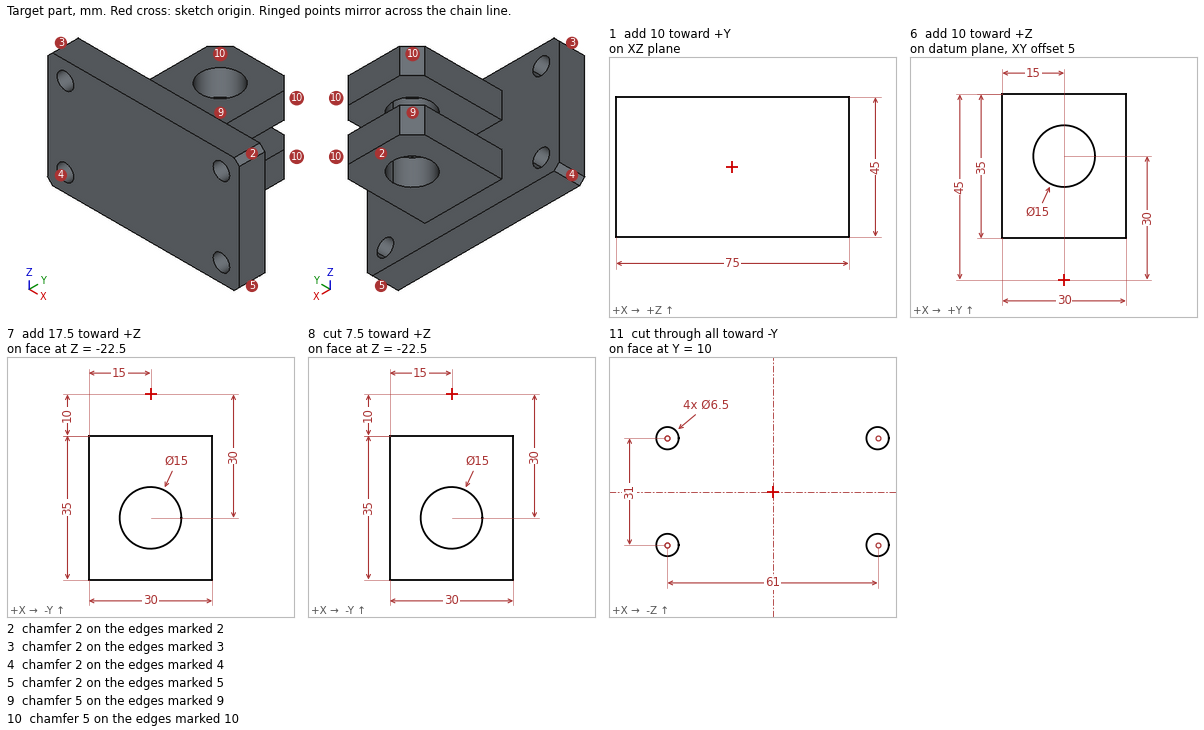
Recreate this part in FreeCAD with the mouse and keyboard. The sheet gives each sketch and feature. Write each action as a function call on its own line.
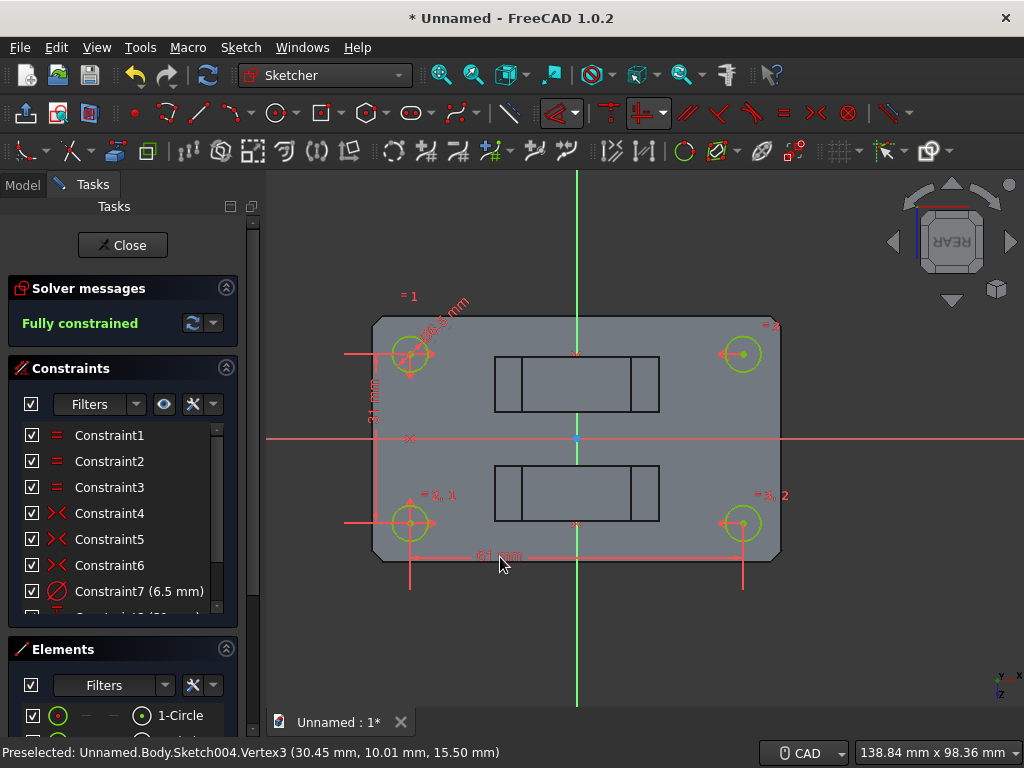
click(123, 245)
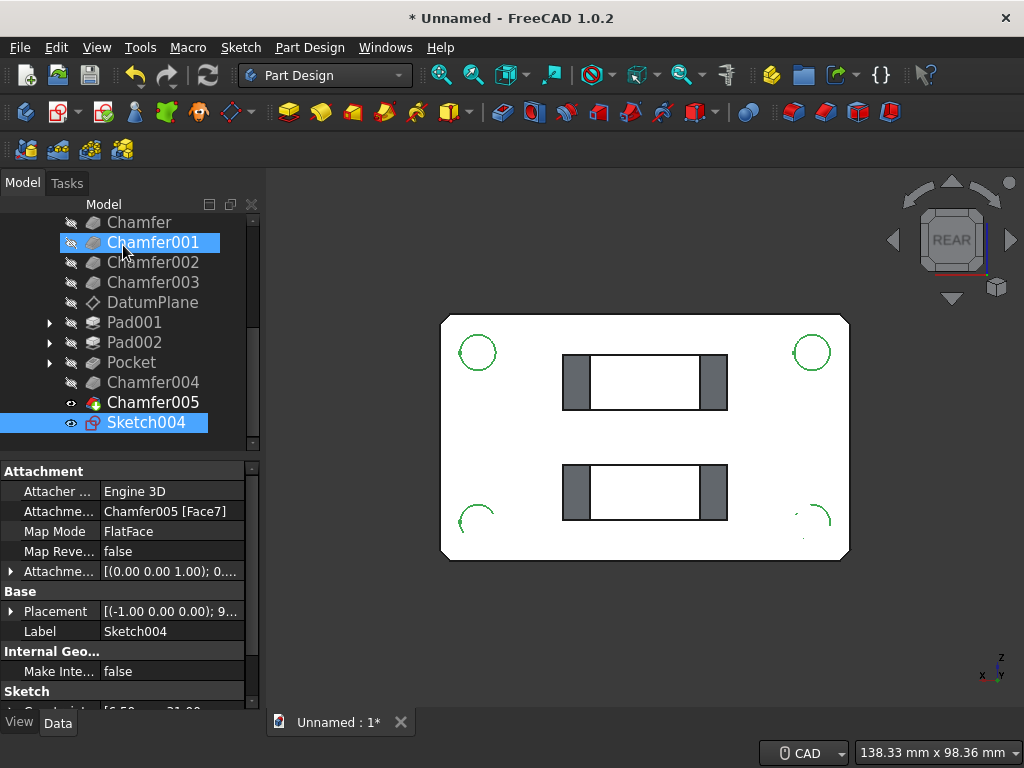
click(504, 112)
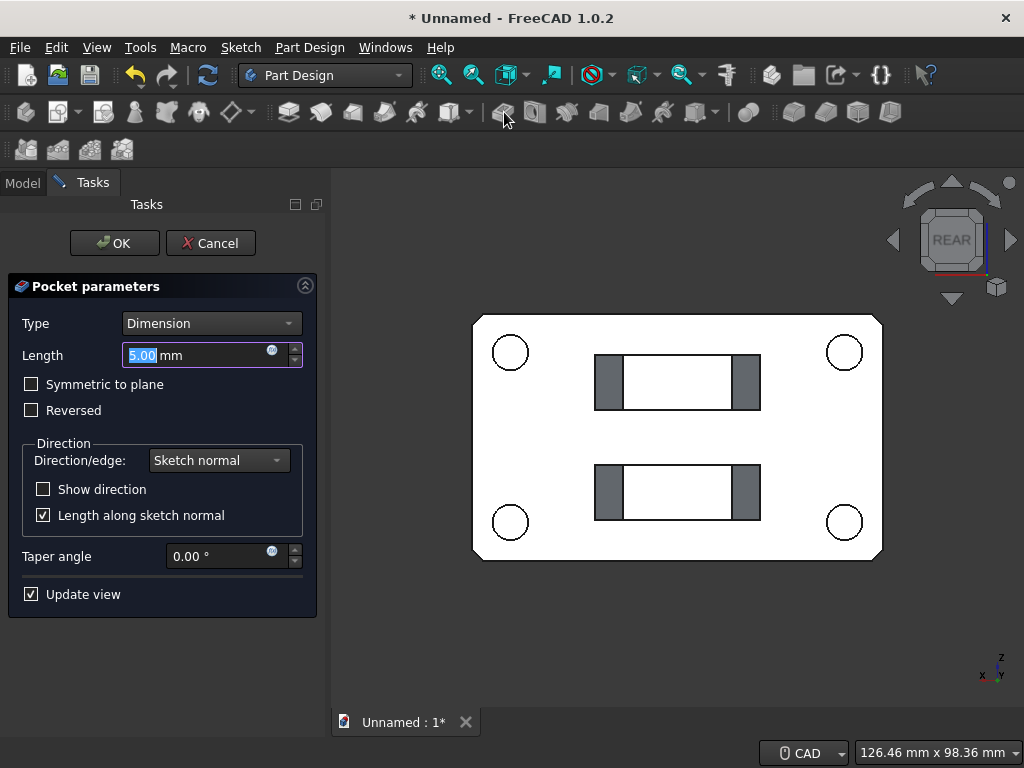
click(212, 324)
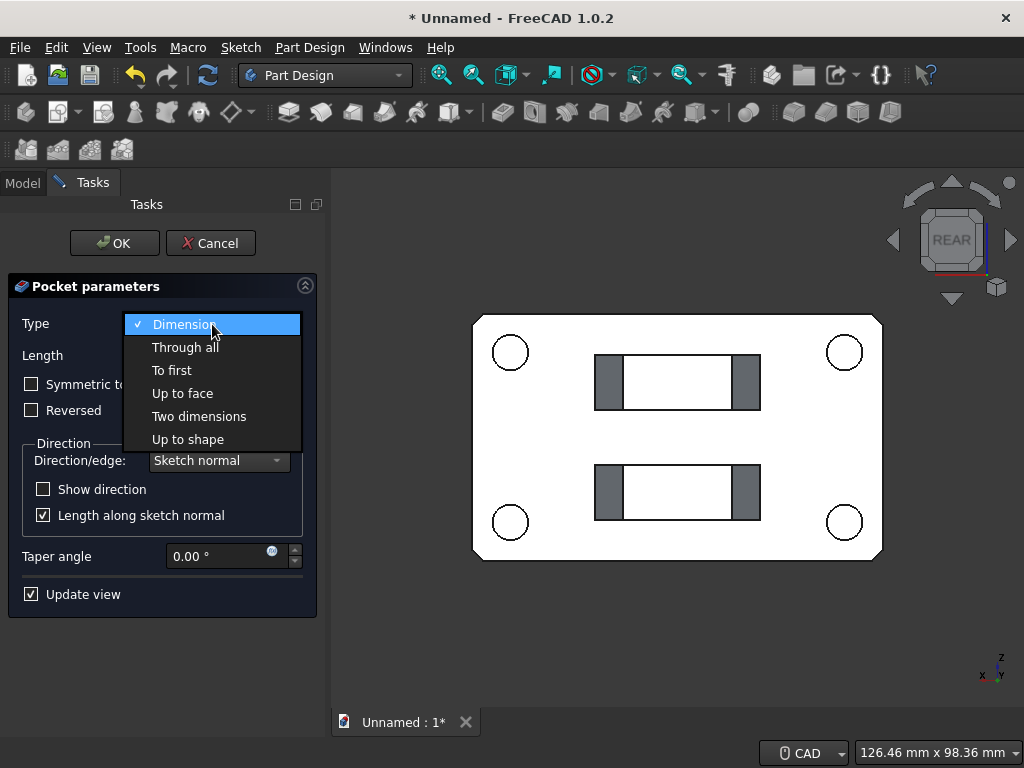
click(212, 348)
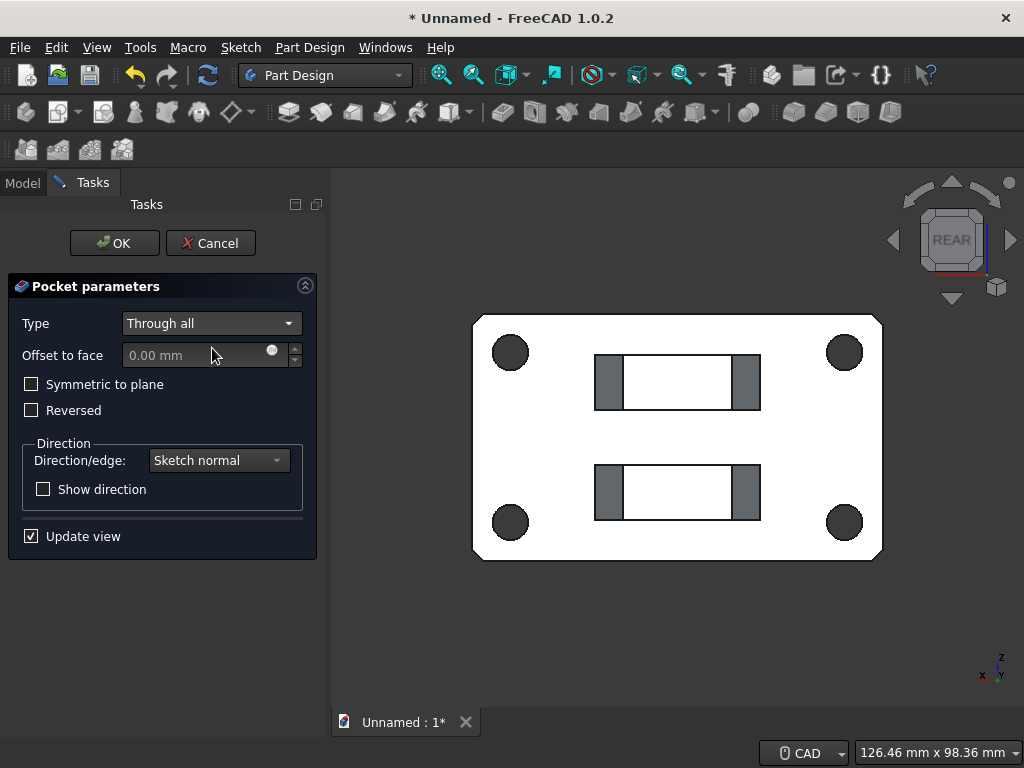
click(115, 243)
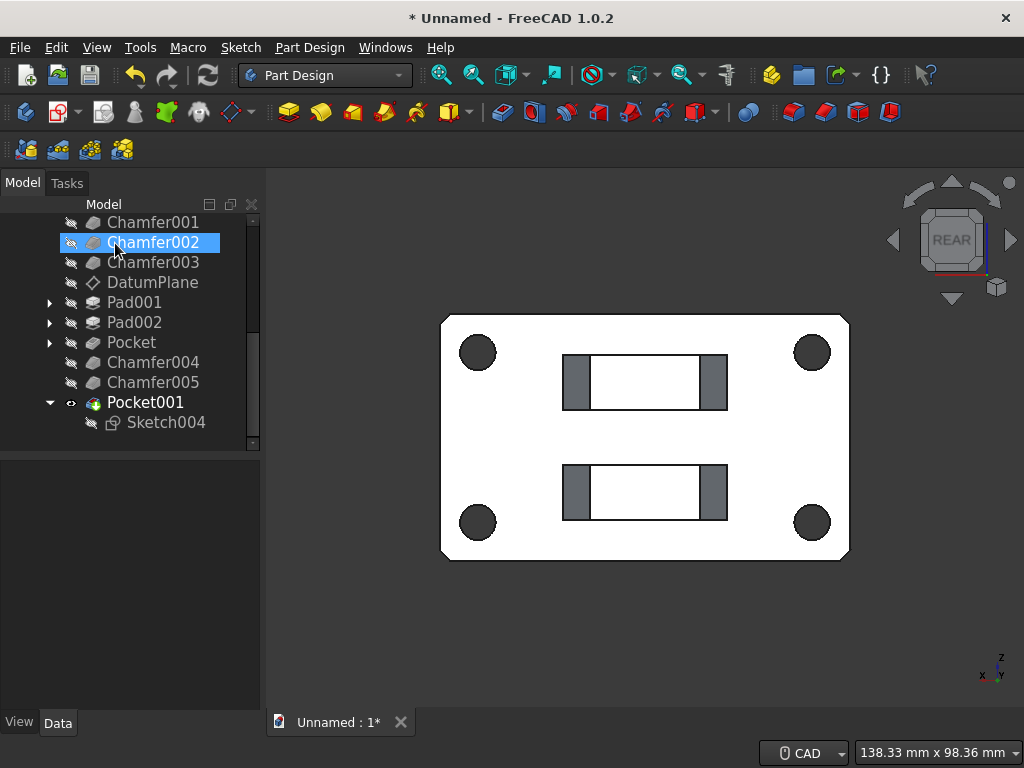
key(0)